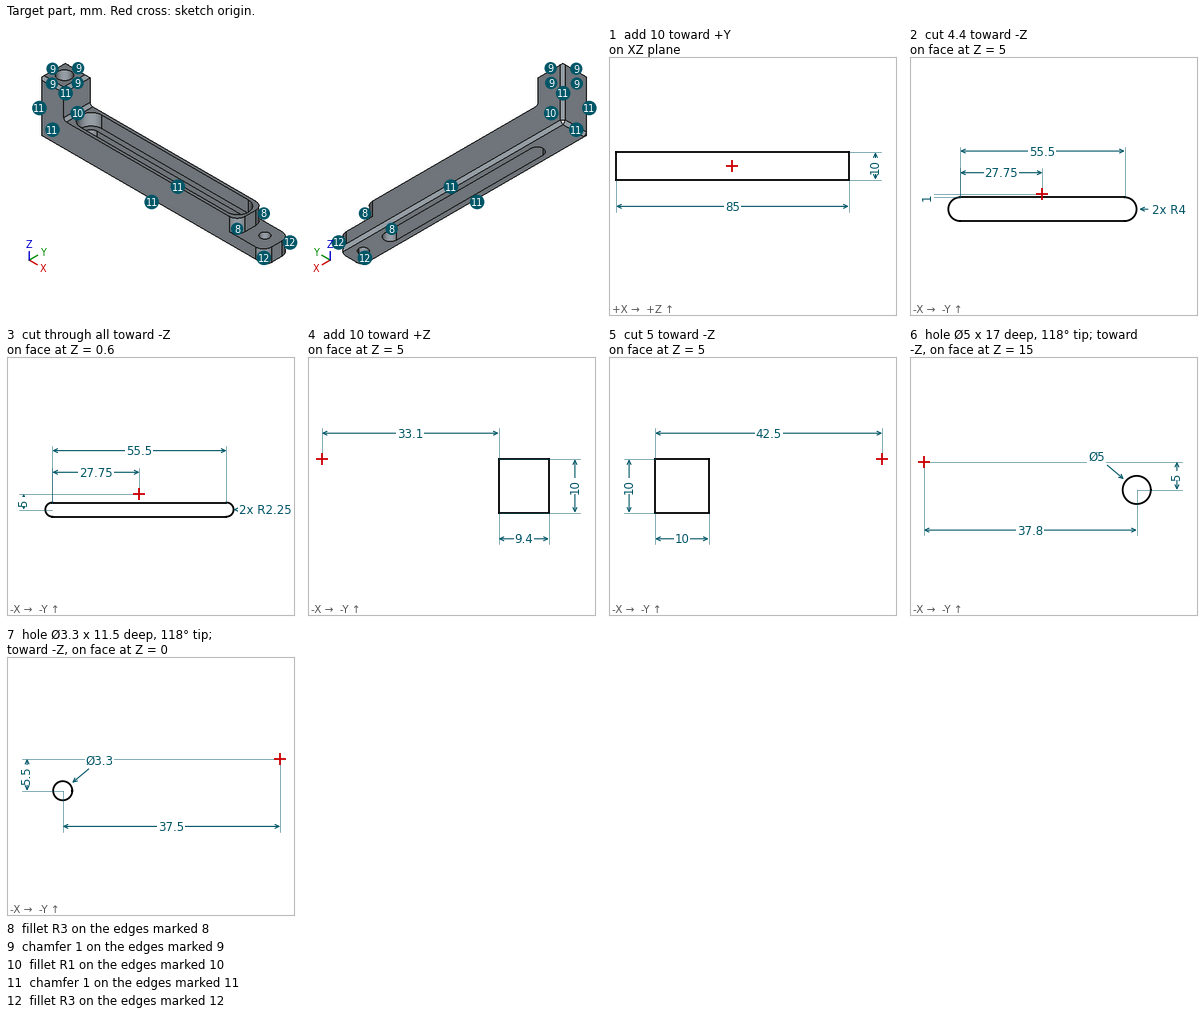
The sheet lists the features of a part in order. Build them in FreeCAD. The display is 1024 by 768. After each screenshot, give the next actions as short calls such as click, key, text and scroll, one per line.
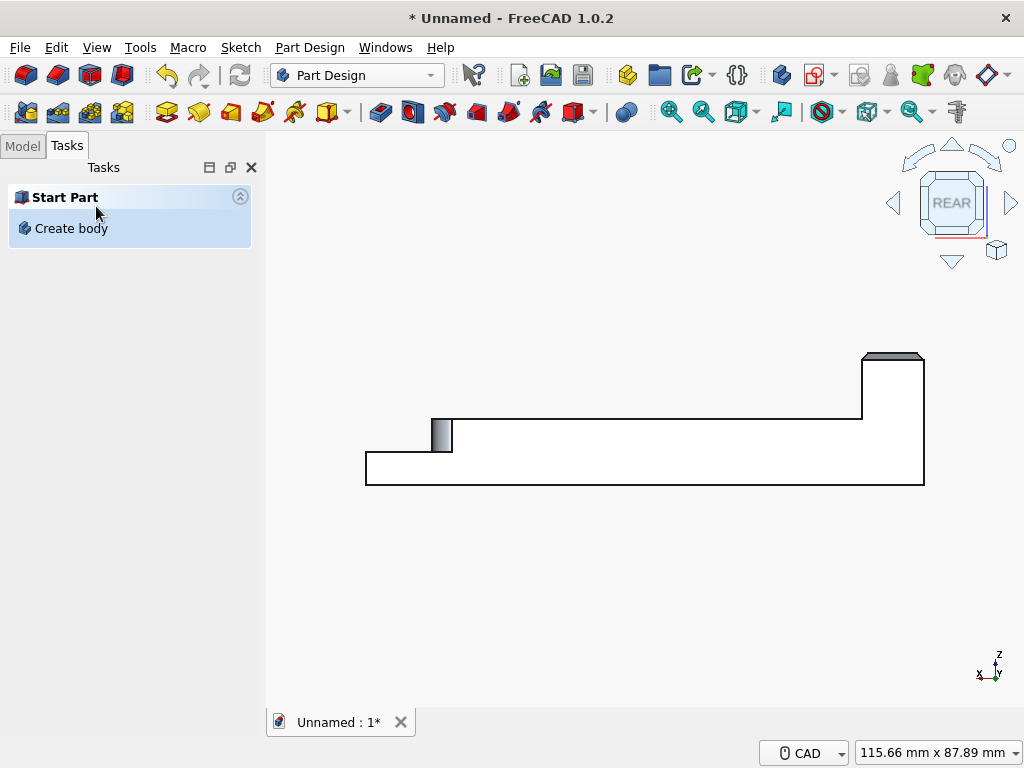
key(6)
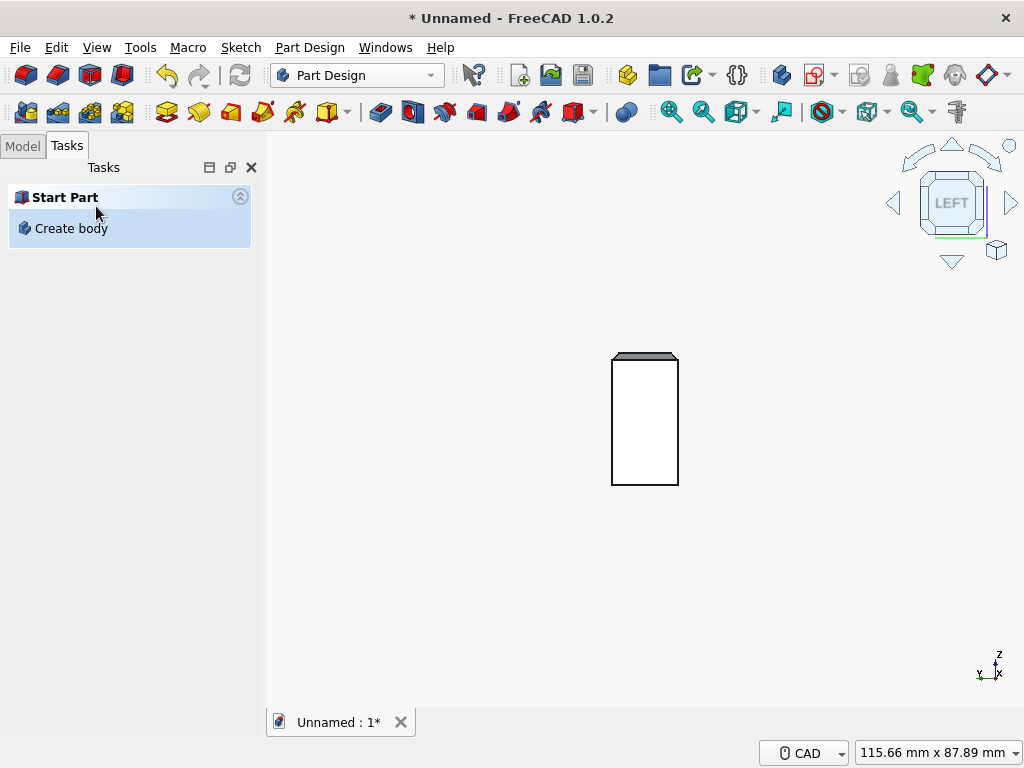
key(v)
key(f)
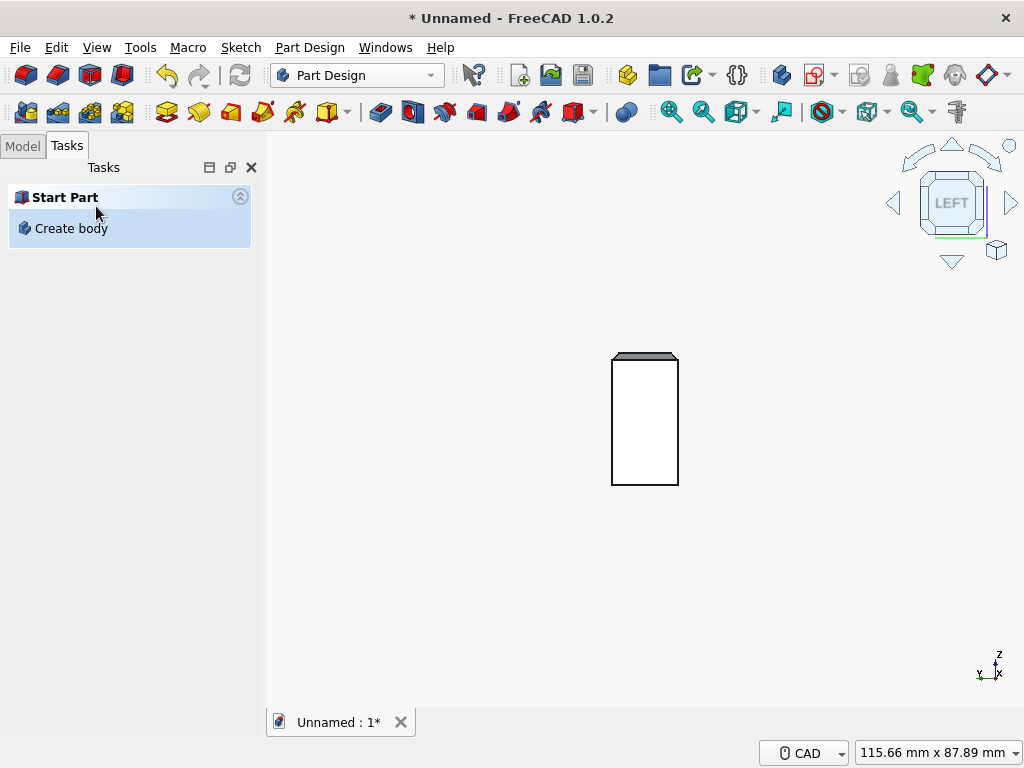
key(v)
key(3)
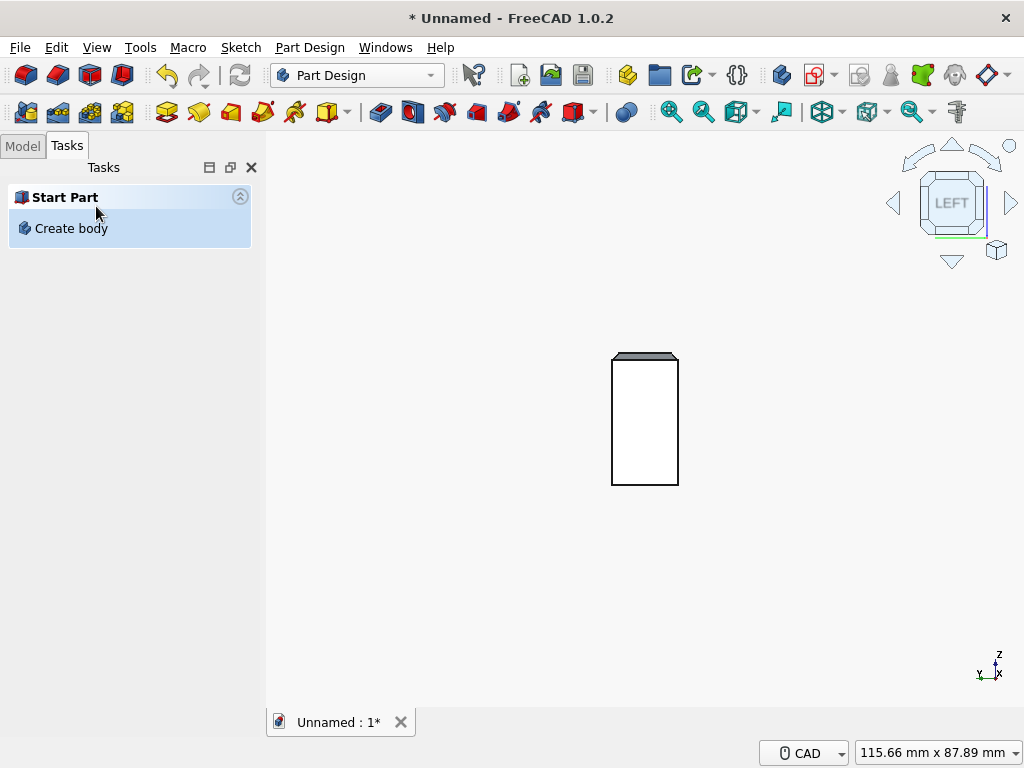
key(0)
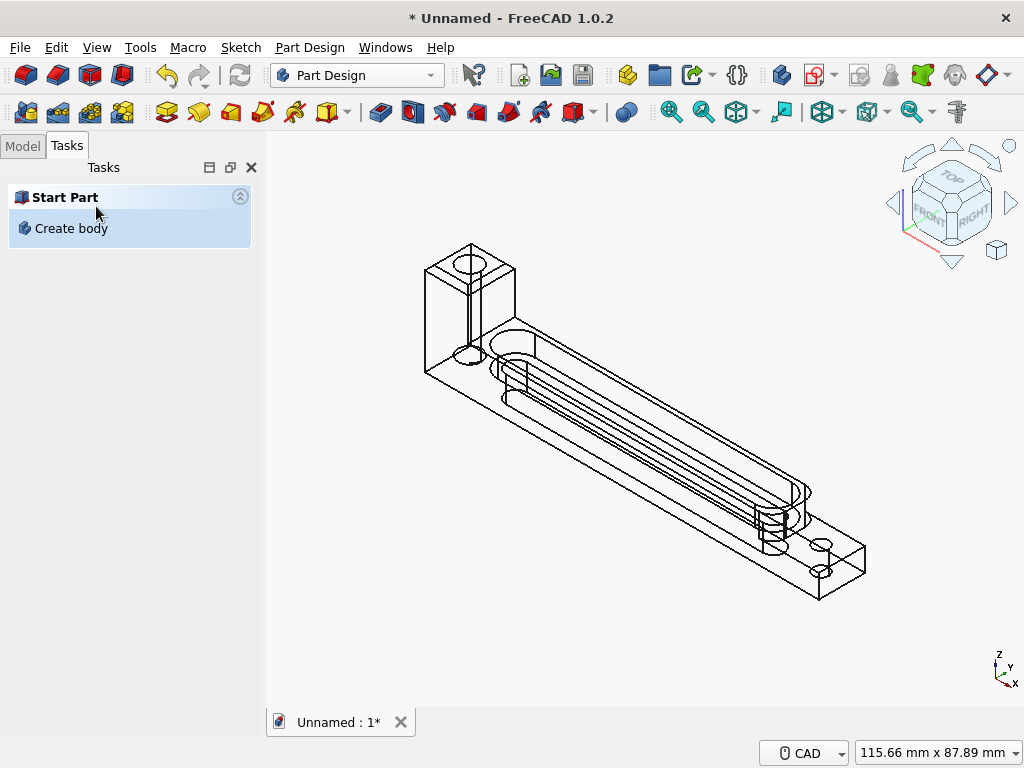
click(492, 329)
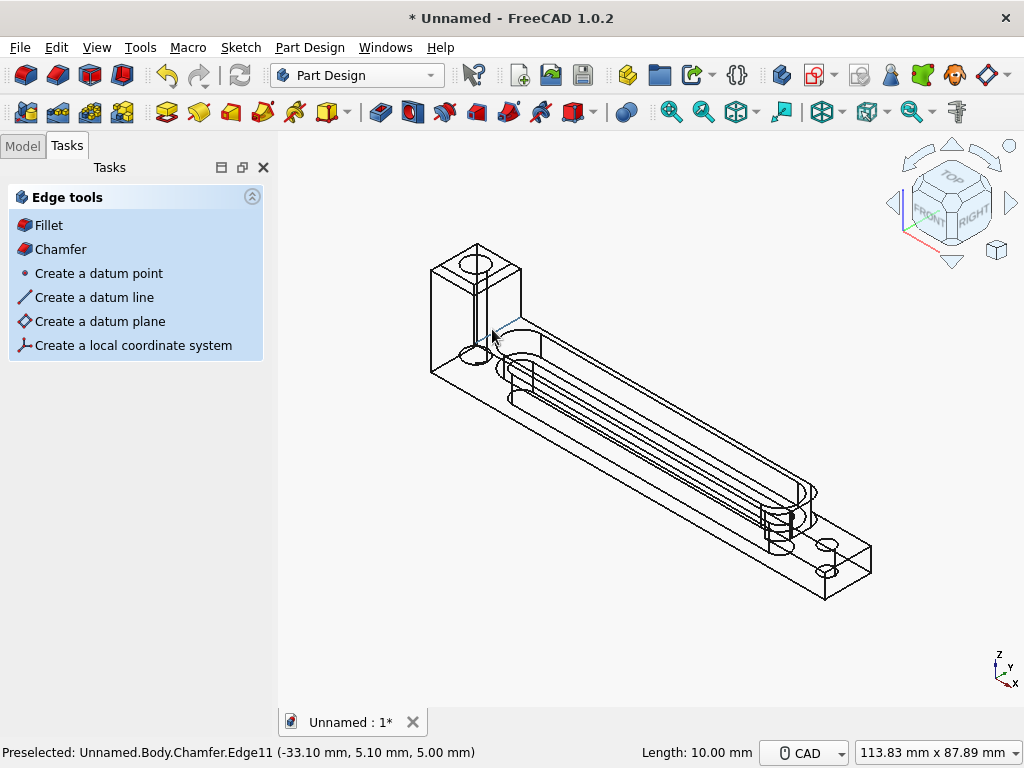
key(v)
key(1)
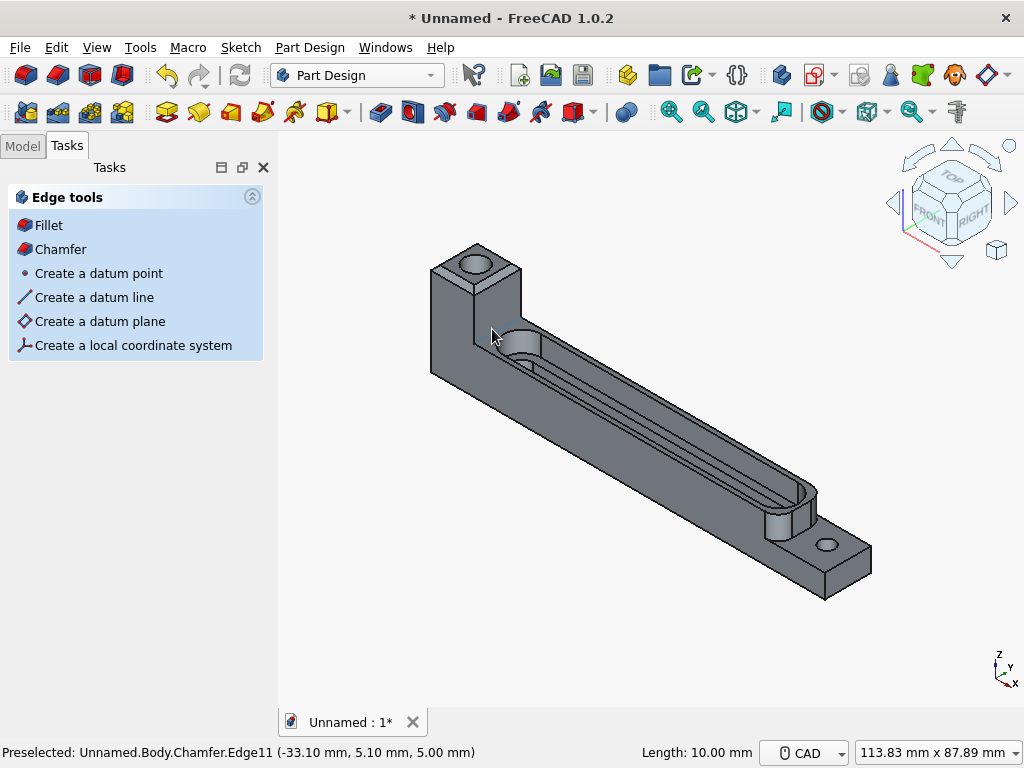
click(26, 76)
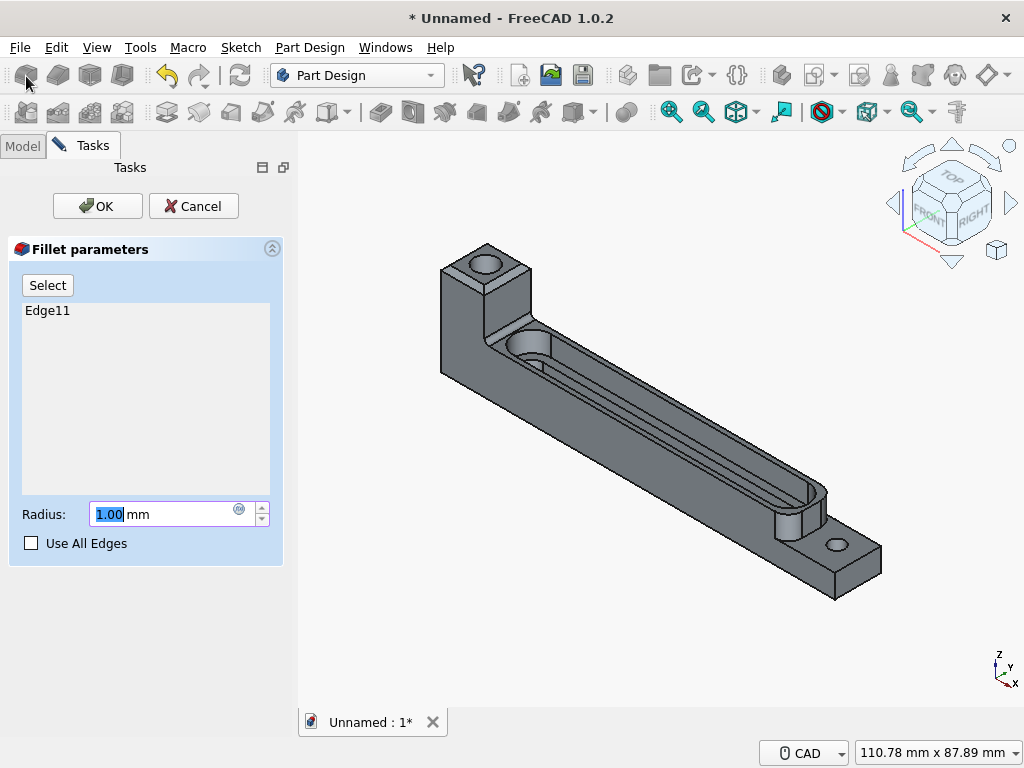
text(1)
key(Tab)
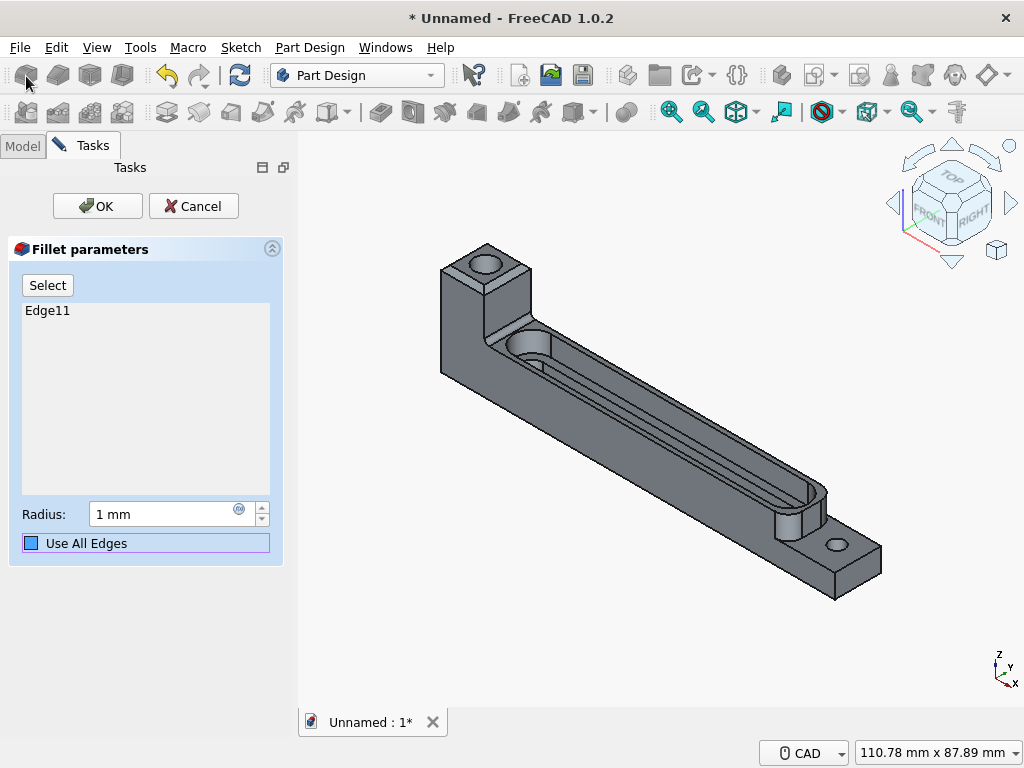
click(98, 206)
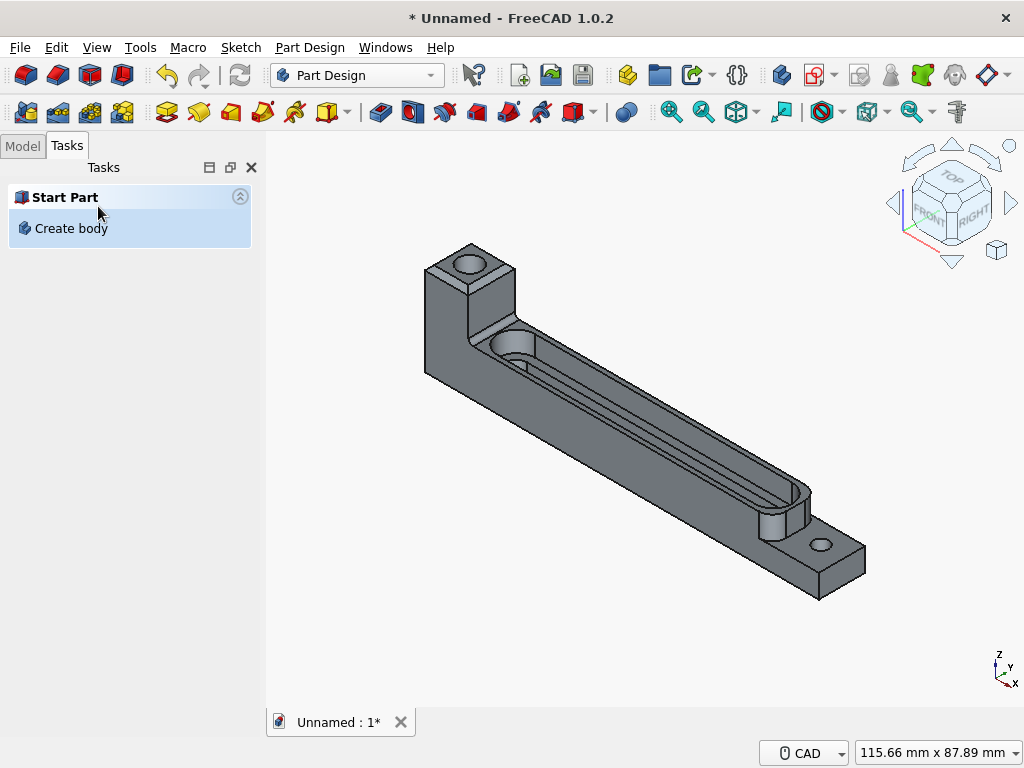
key(2)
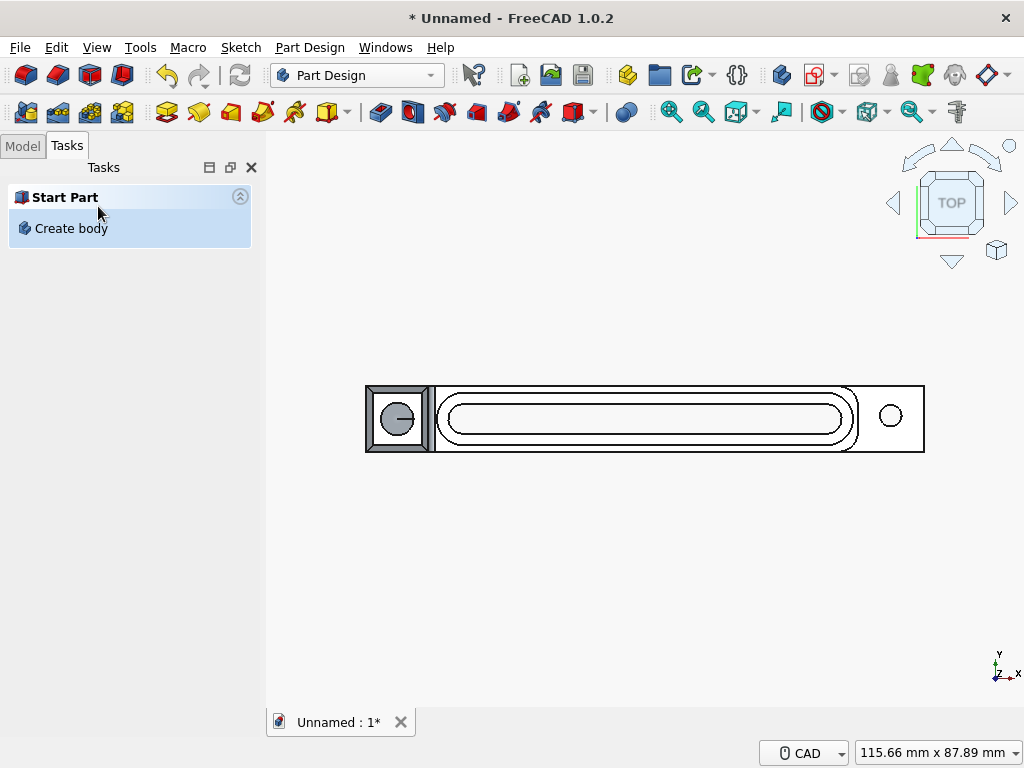
key(0)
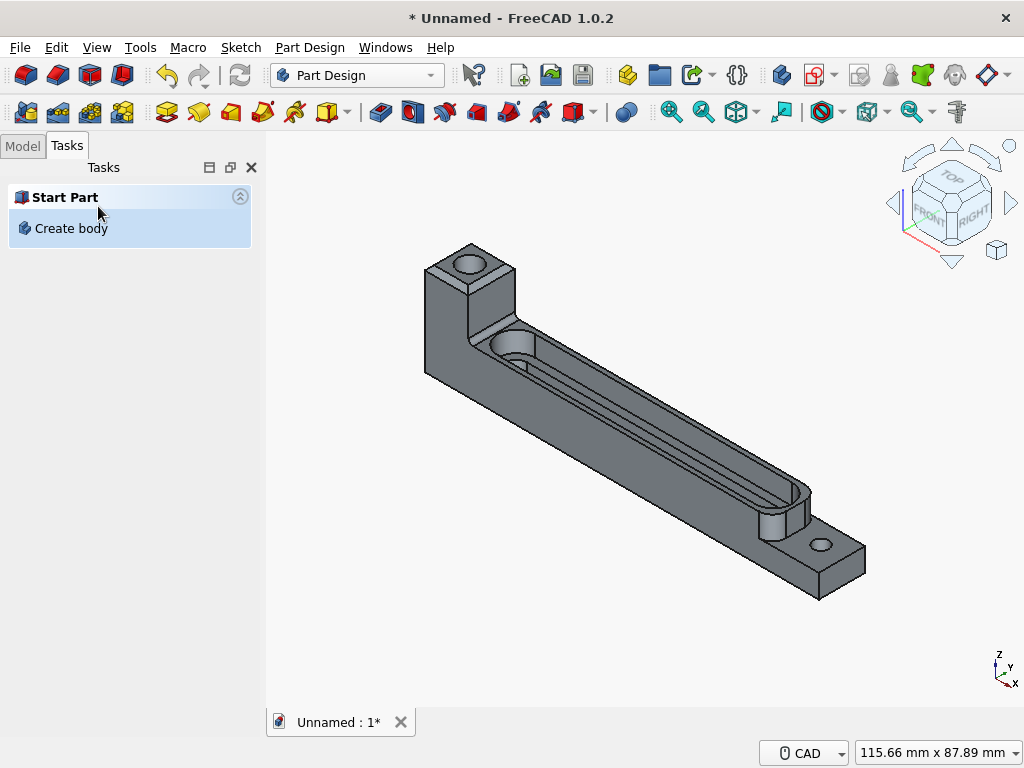
key(1)